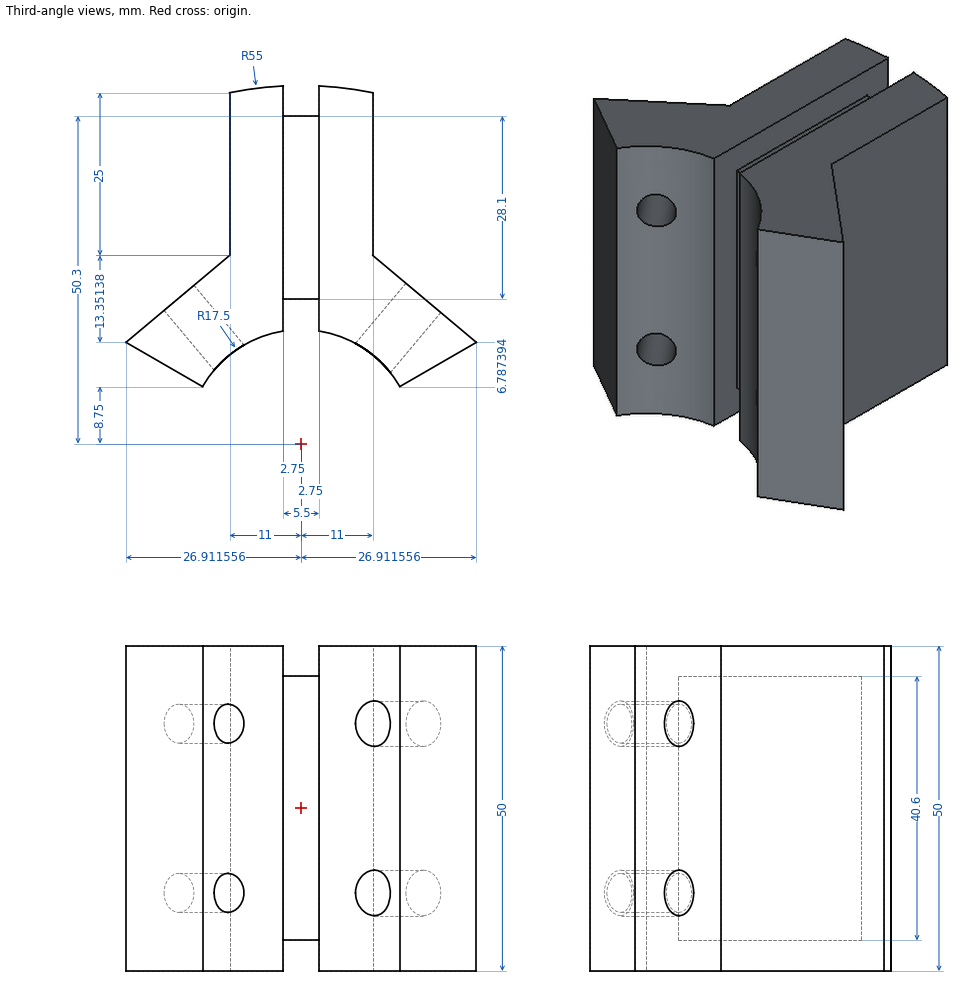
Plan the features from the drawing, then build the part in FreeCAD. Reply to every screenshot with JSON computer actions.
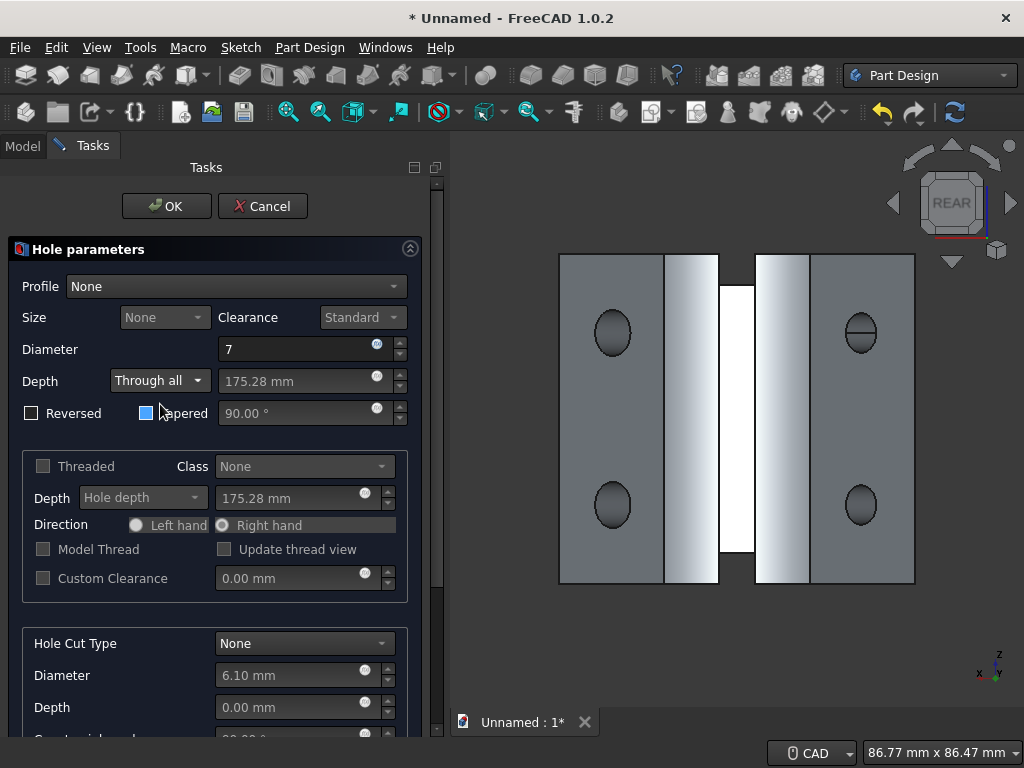
{"action": "left_click", "coordinate": [167, 206]}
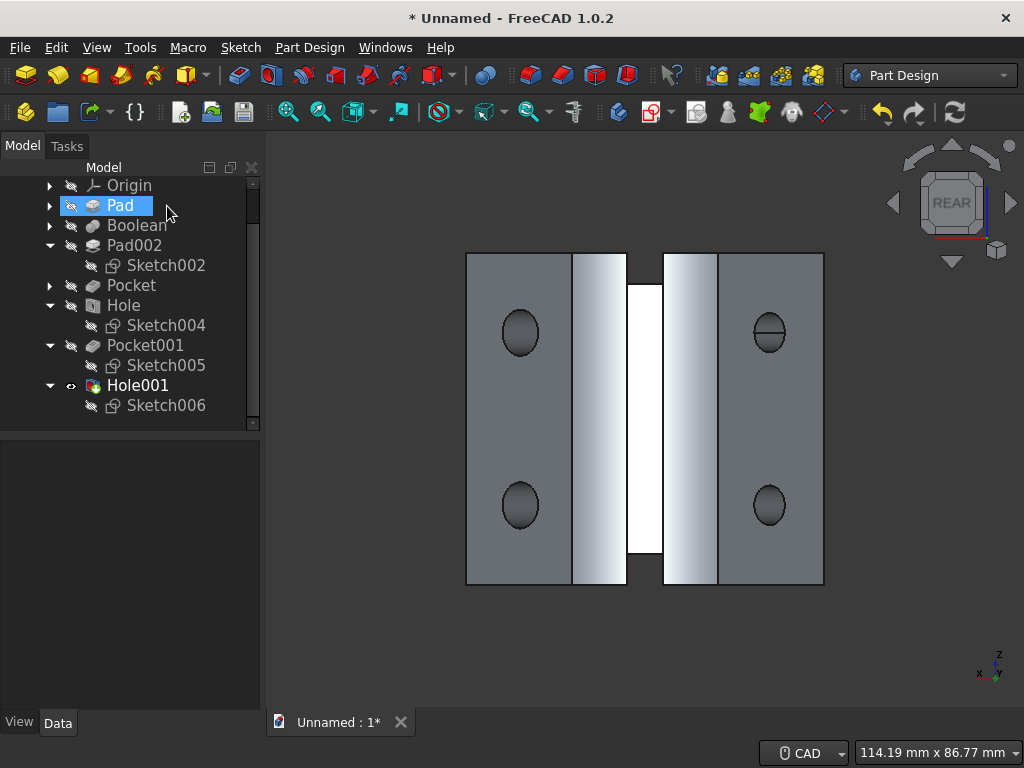
{"action": "key", "text": "0"}